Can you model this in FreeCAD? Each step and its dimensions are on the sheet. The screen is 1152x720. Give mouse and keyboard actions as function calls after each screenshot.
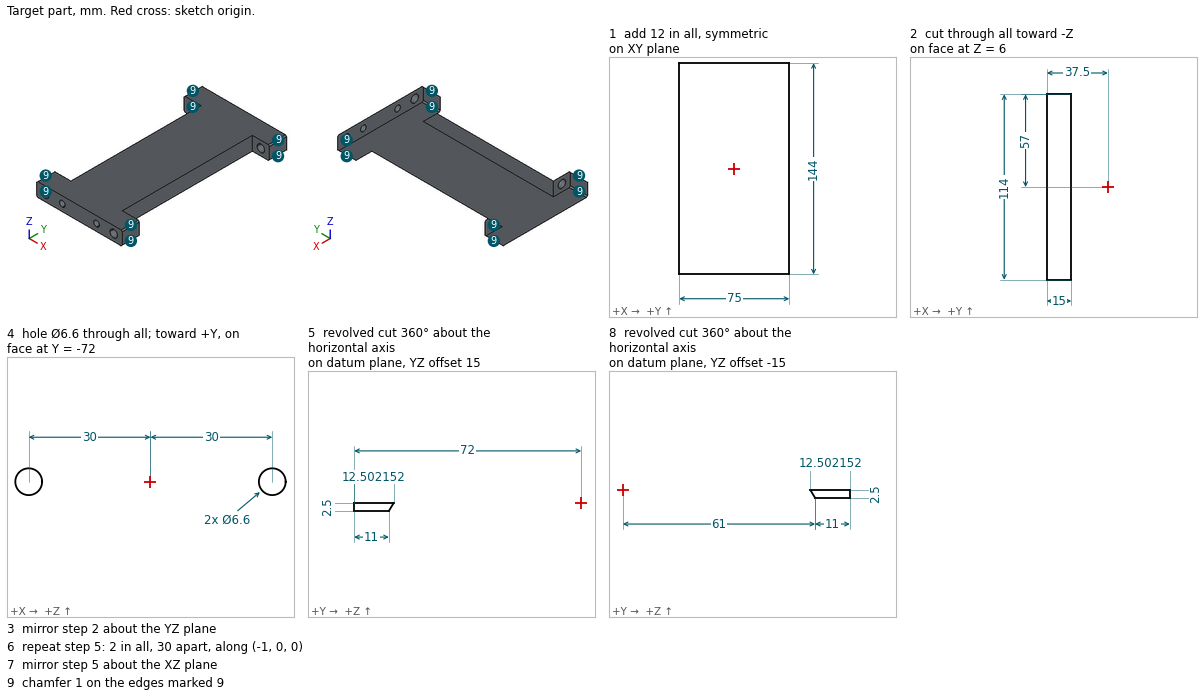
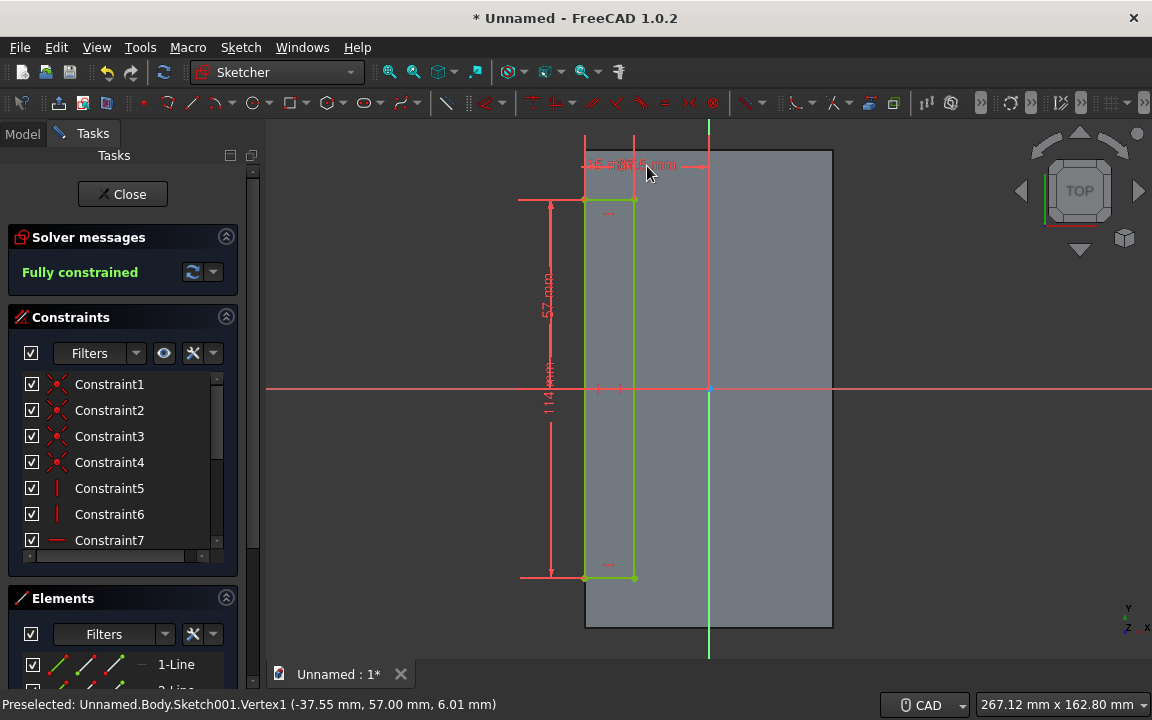
click(123, 194)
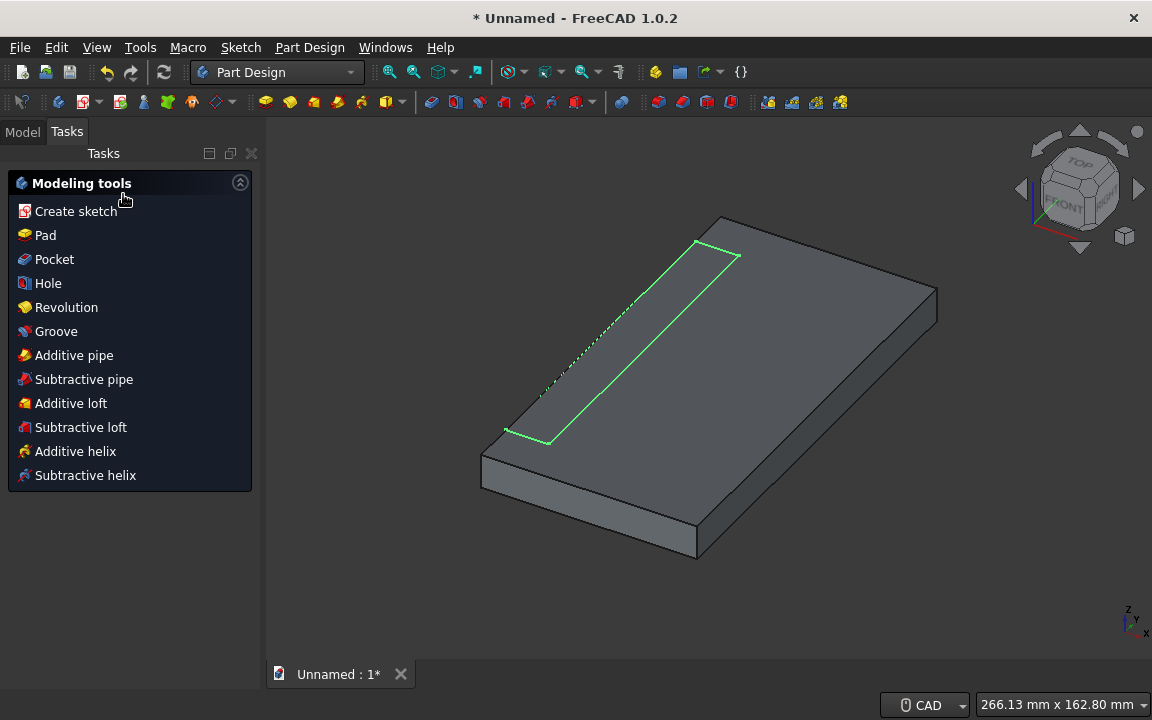
click(432, 102)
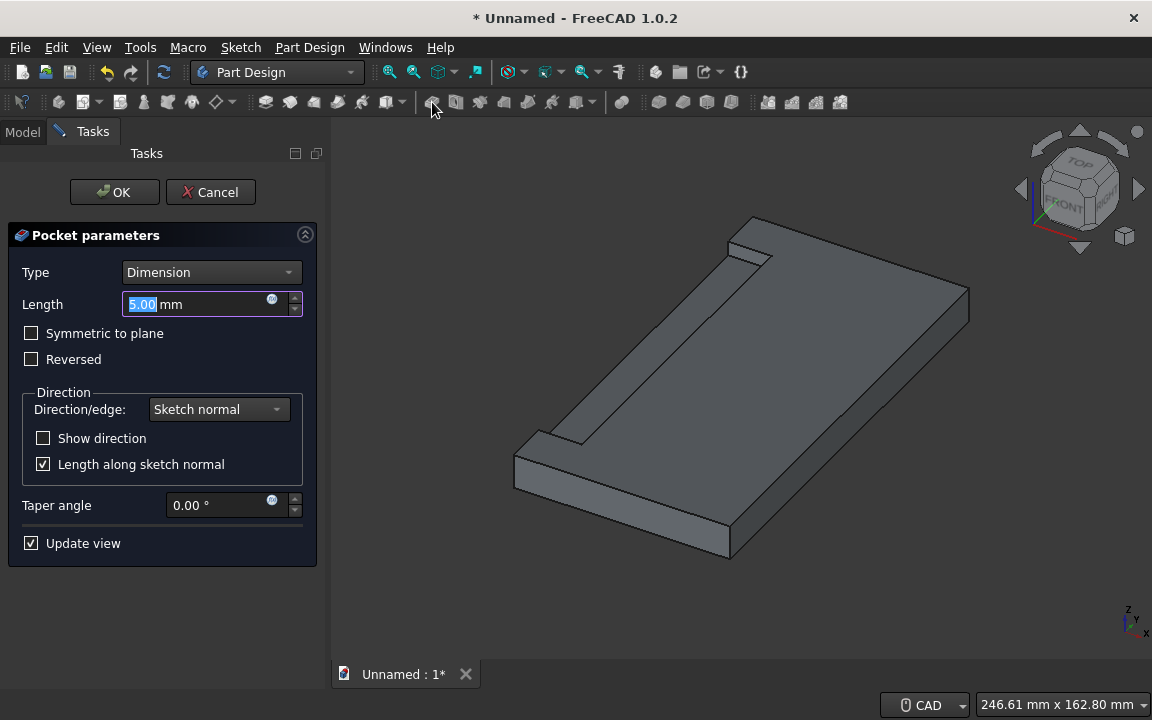
click(212, 272)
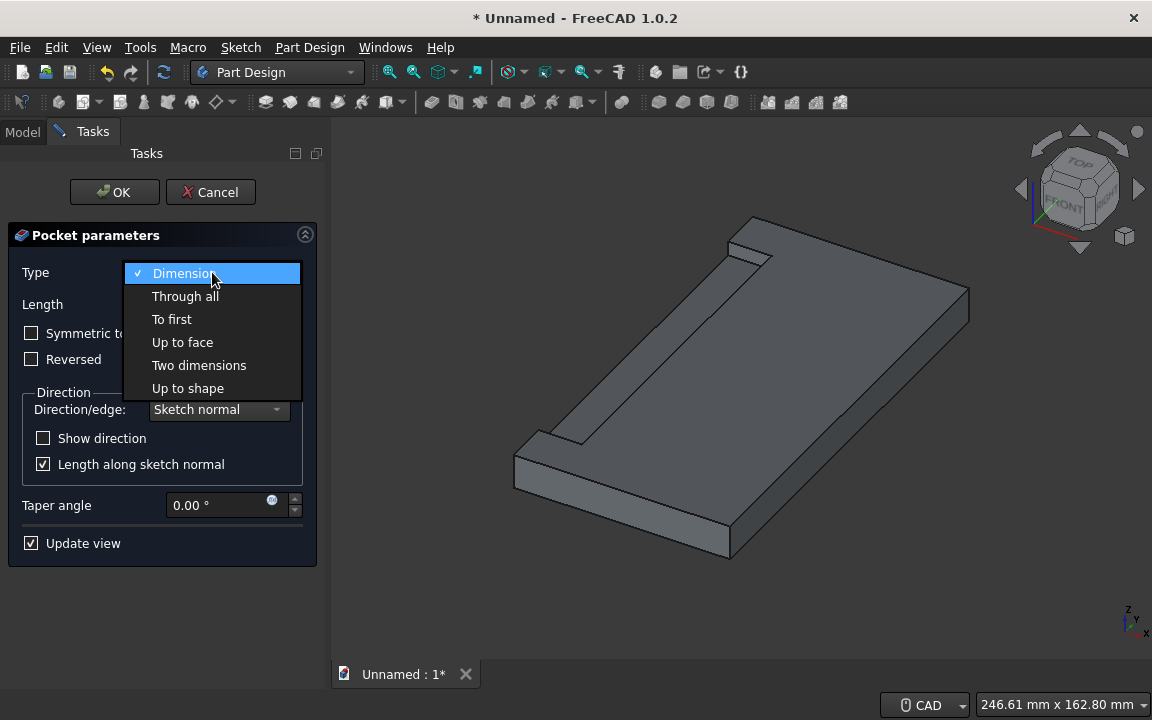
click(212, 296)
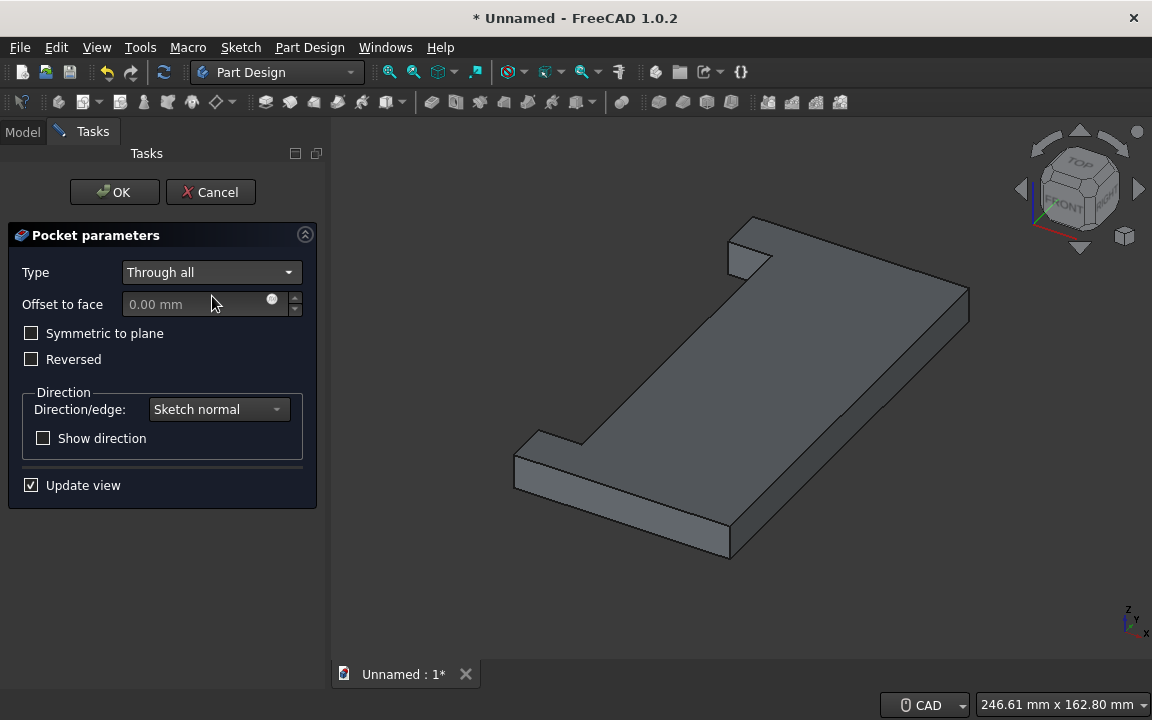
click(115, 192)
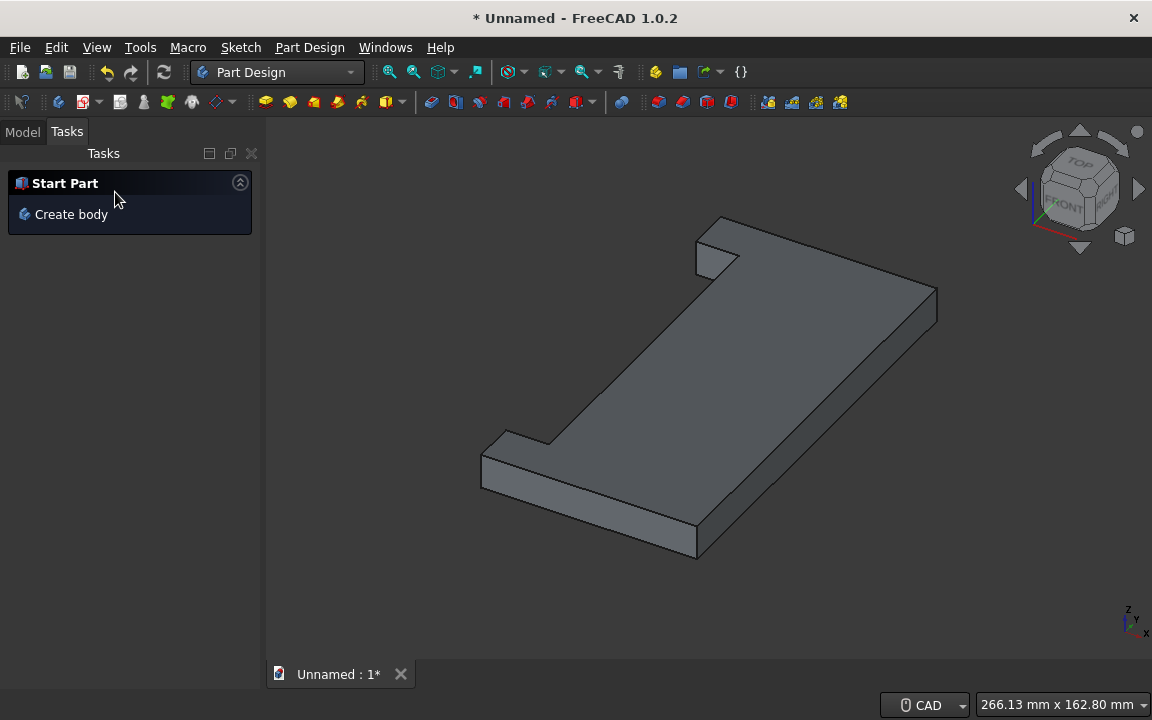
click(23, 131)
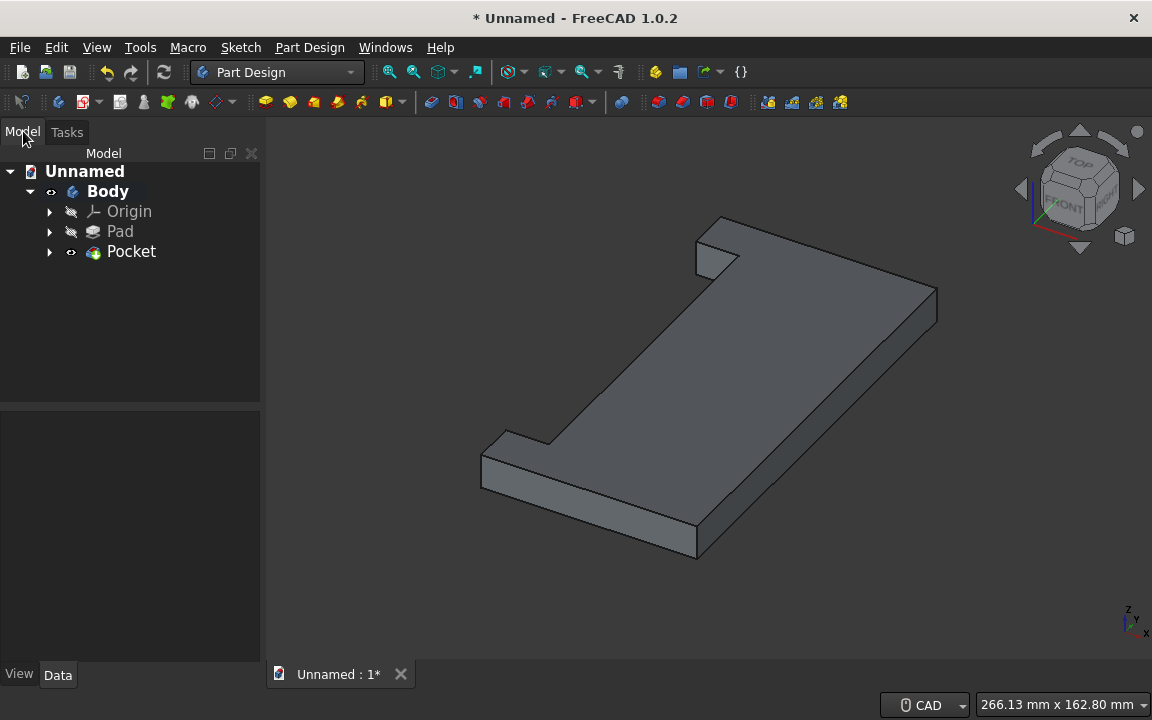
click(116, 252)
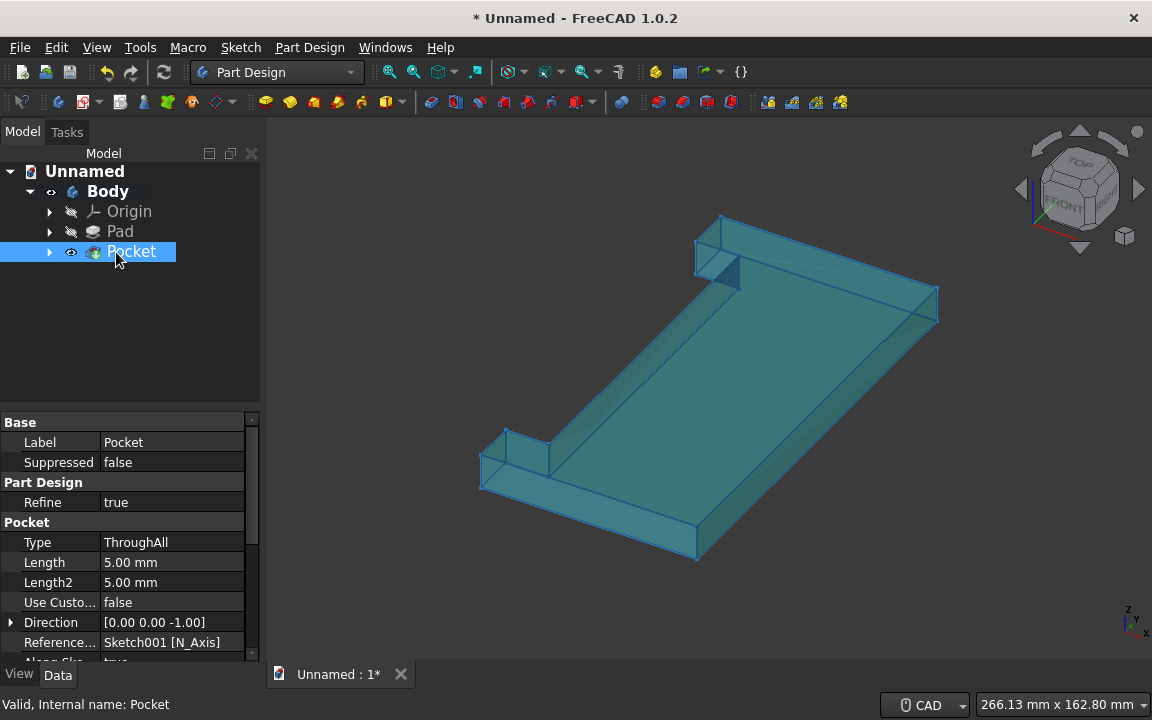
click(768, 102)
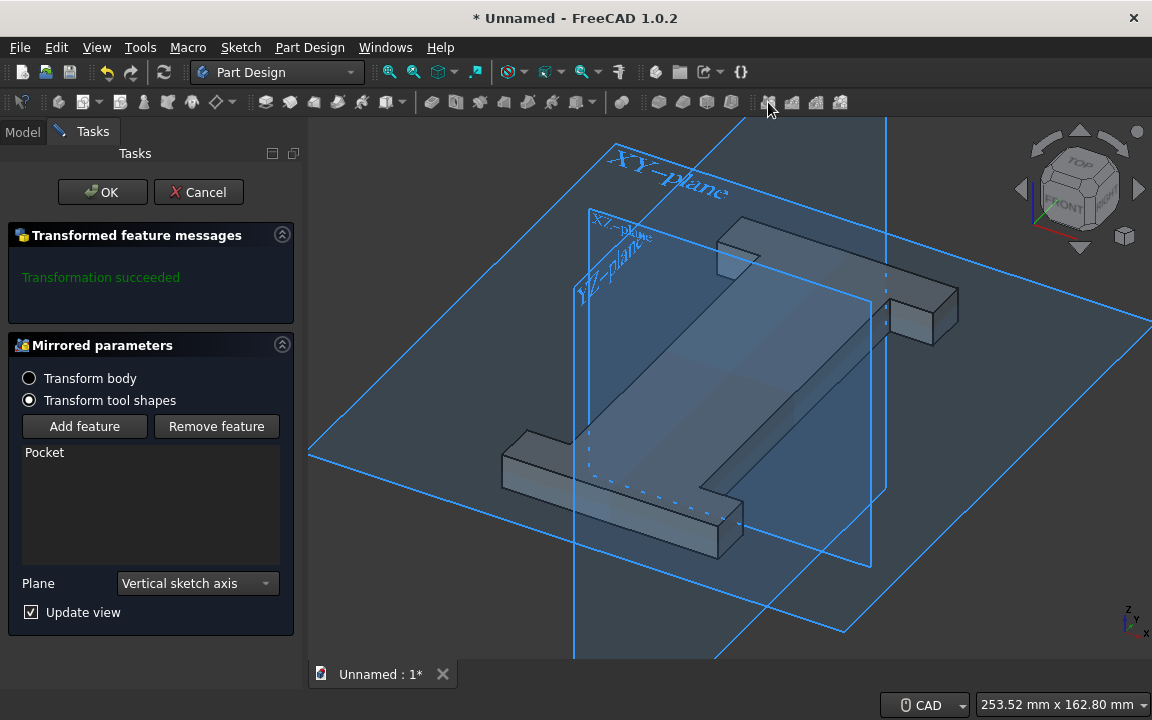
click(198, 584)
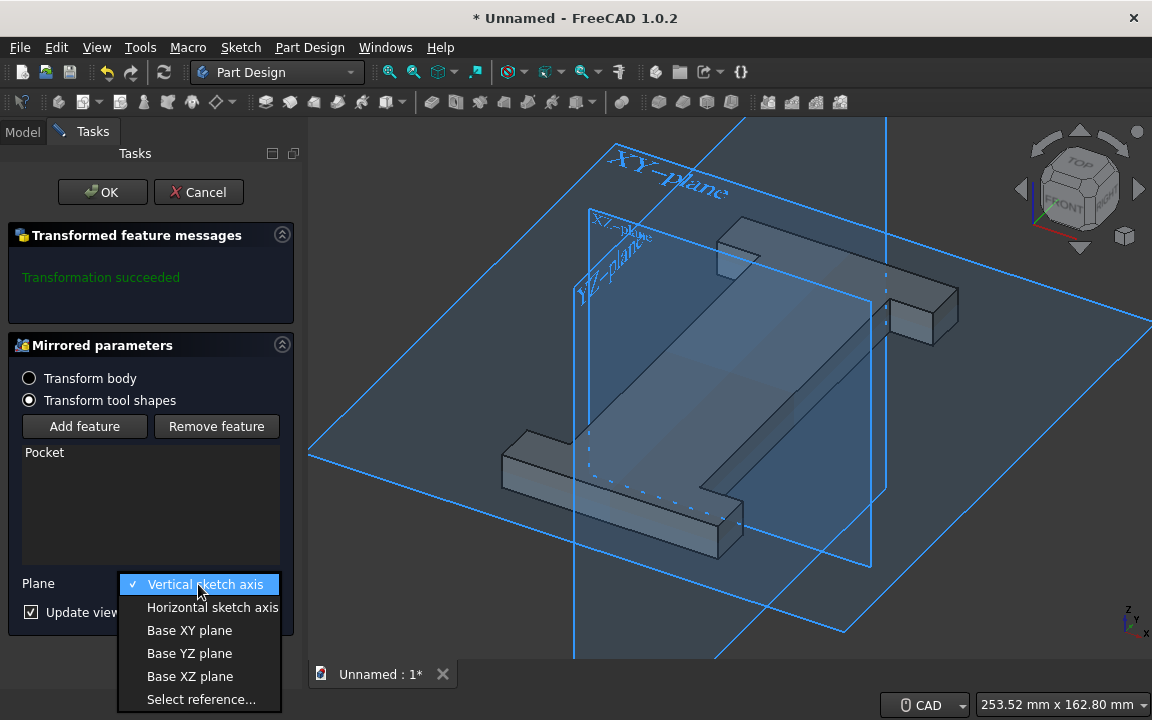
click(198, 654)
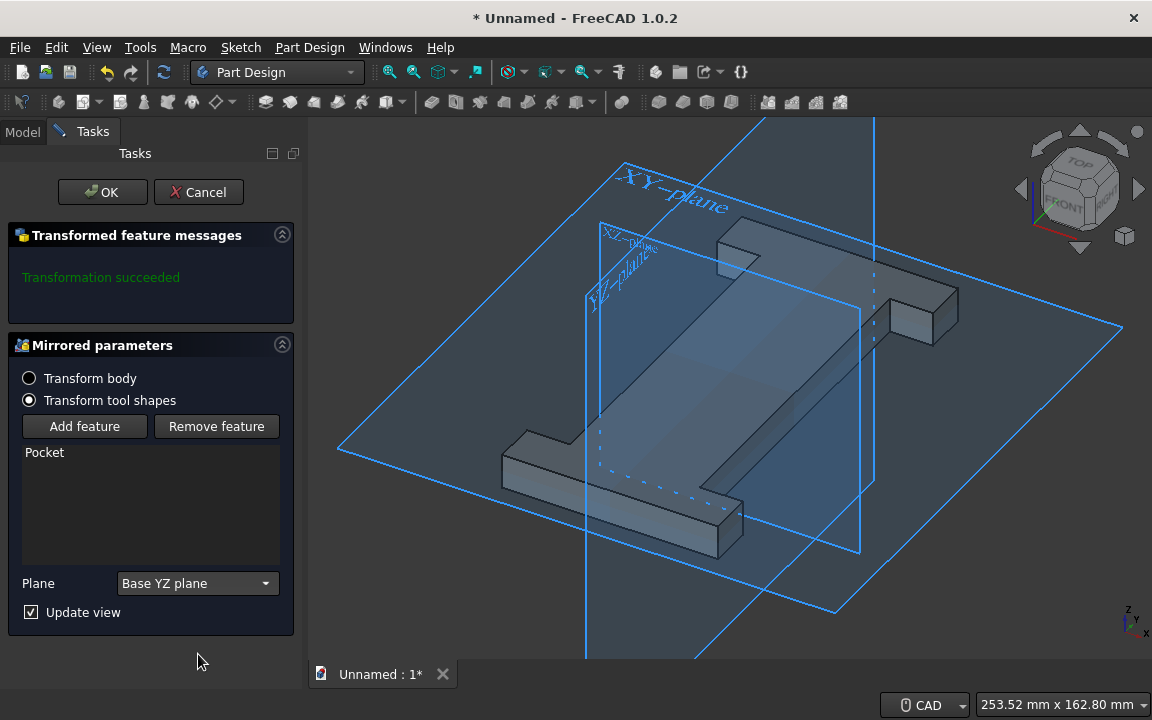
click(103, 192)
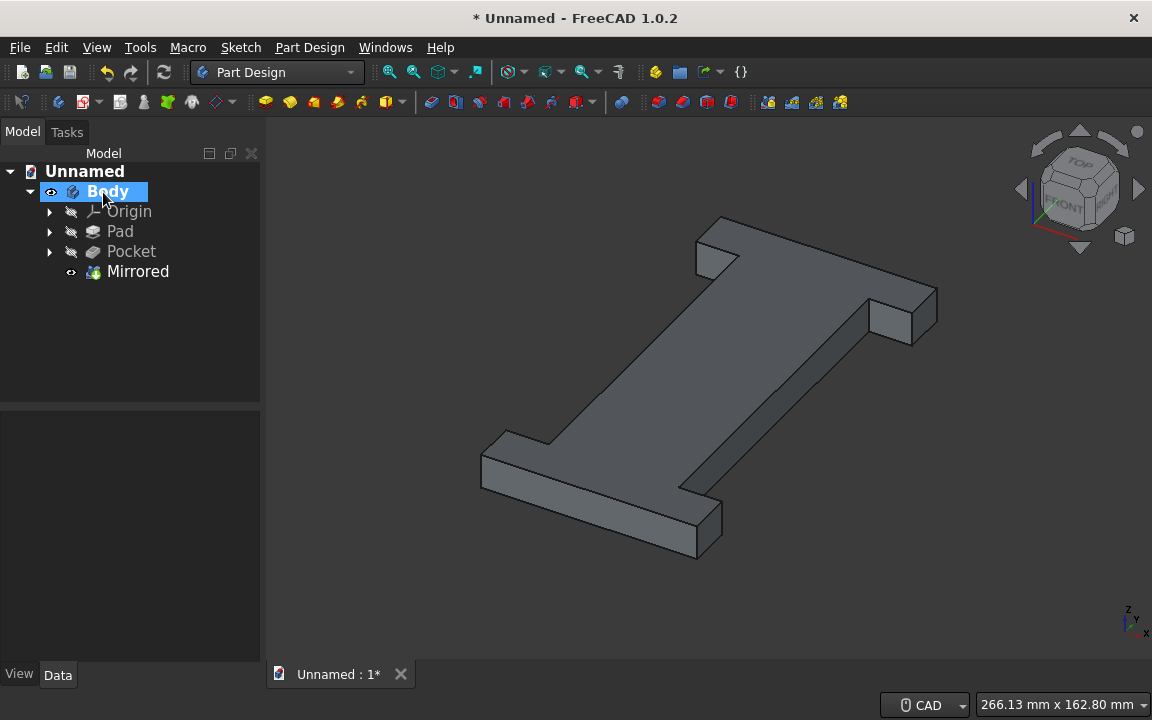
click(651, 527)